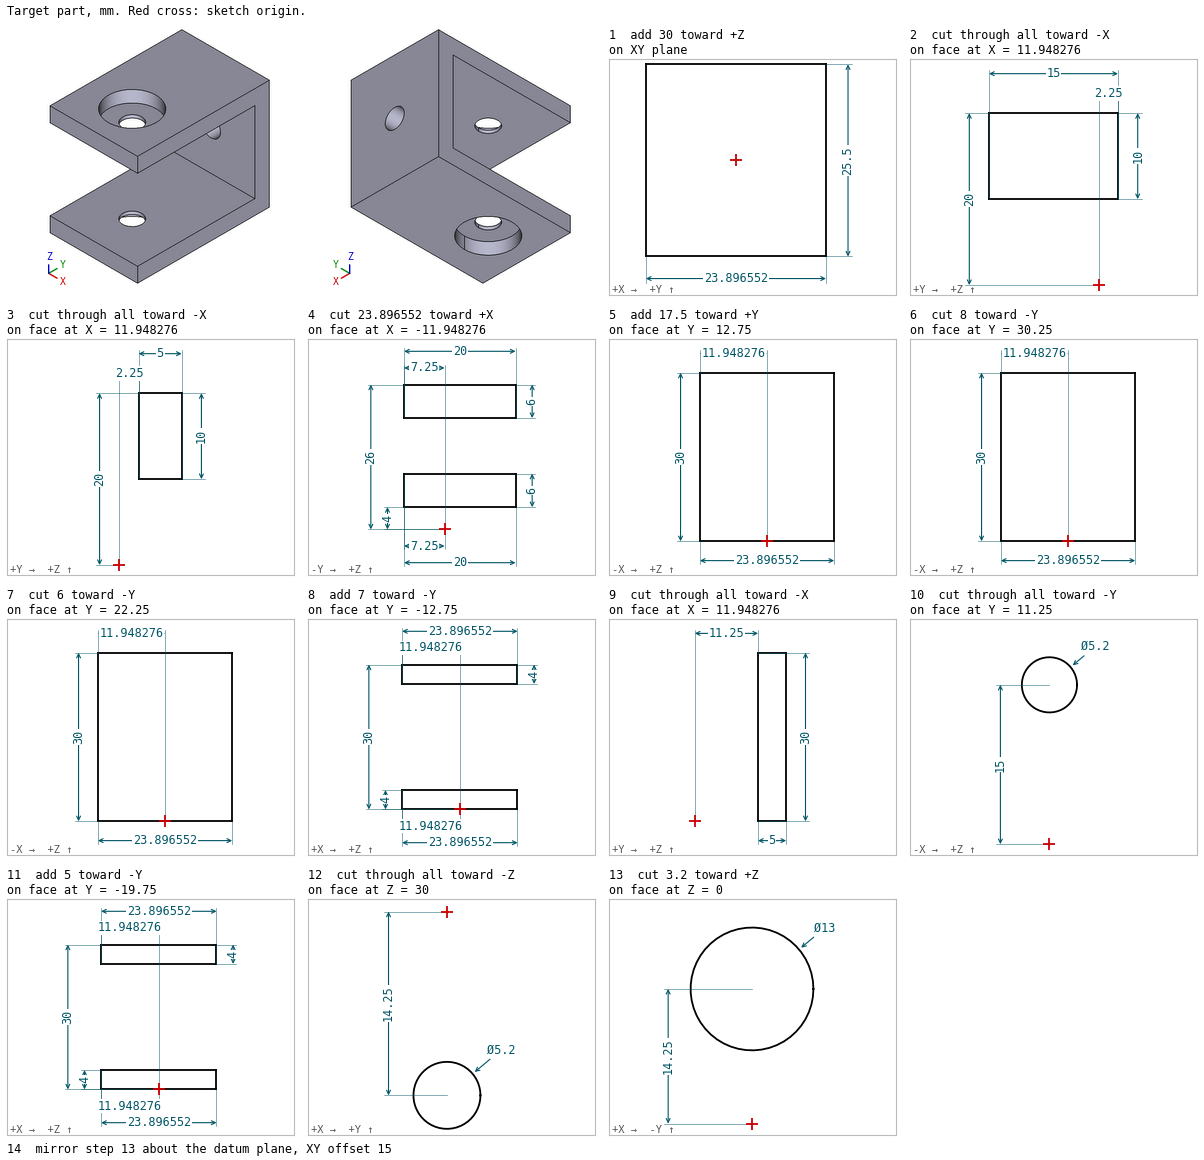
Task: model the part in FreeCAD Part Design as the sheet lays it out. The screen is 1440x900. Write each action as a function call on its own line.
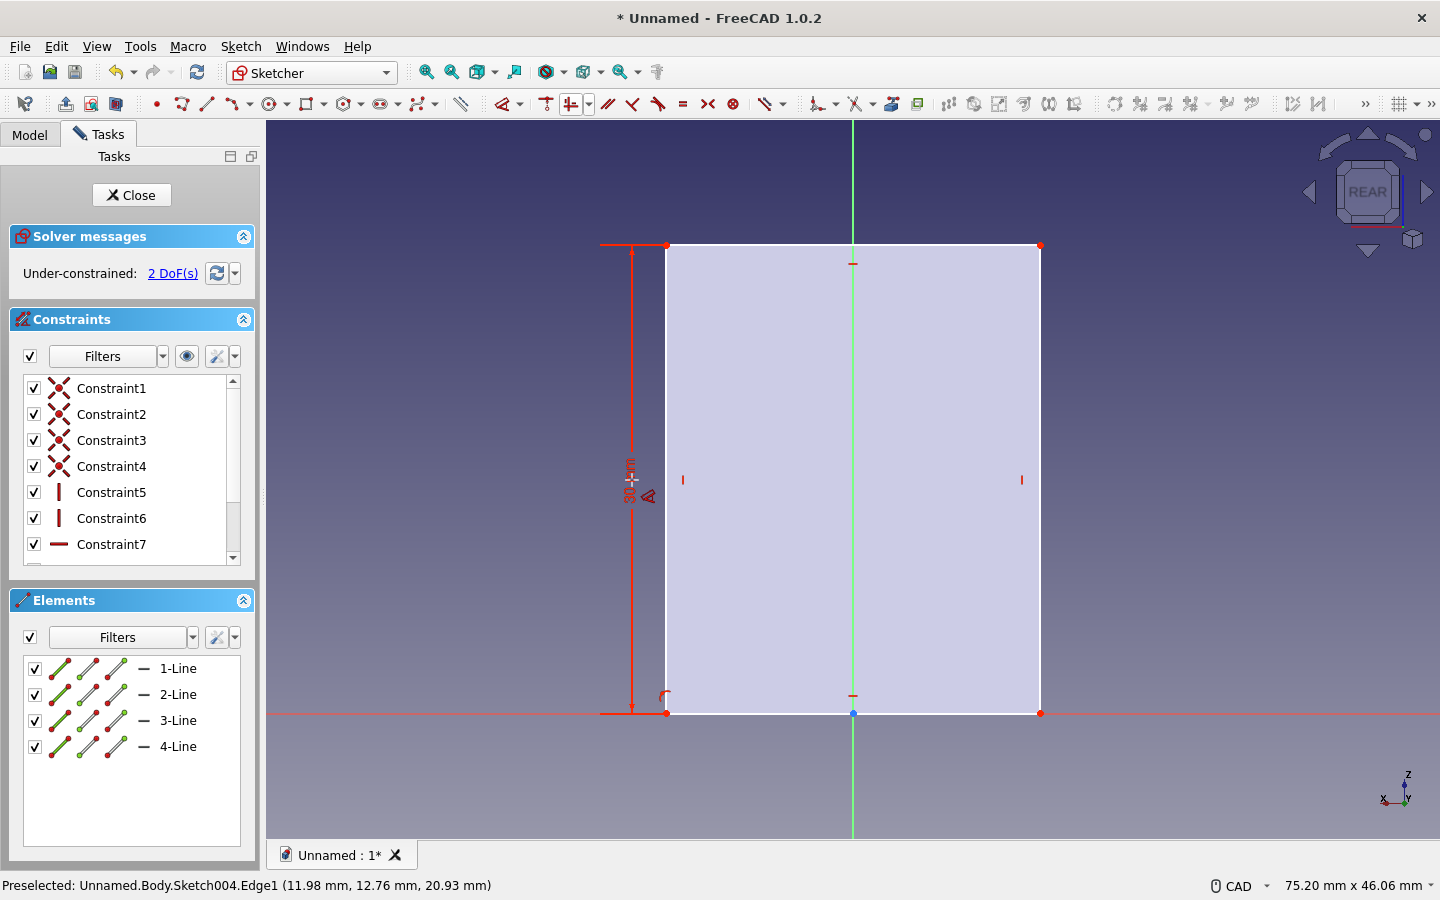
click(778, 714)
click(767, 748)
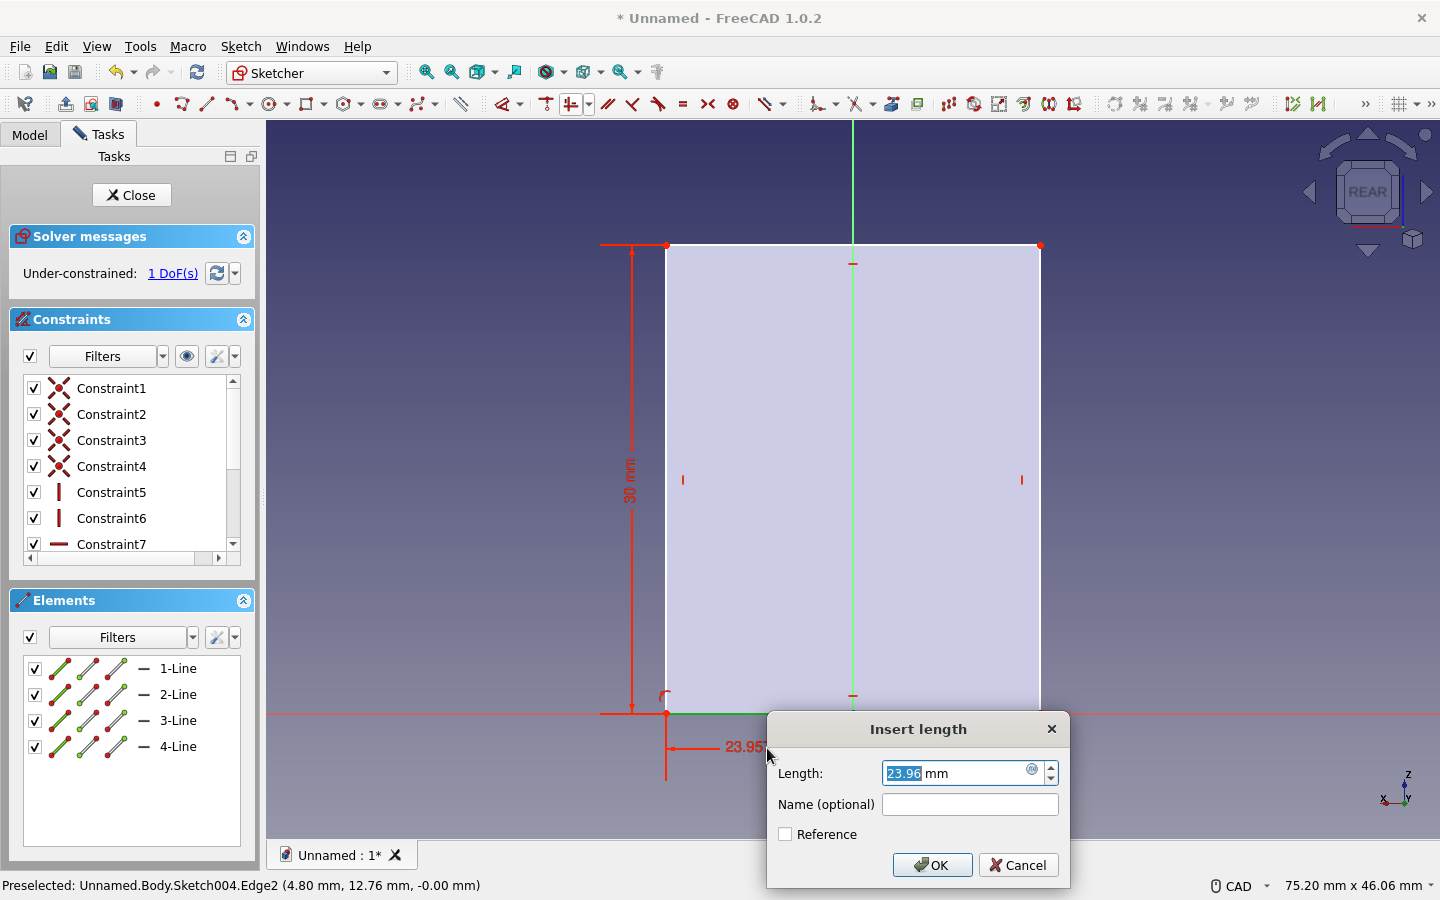
text(23.896552)
key(Return)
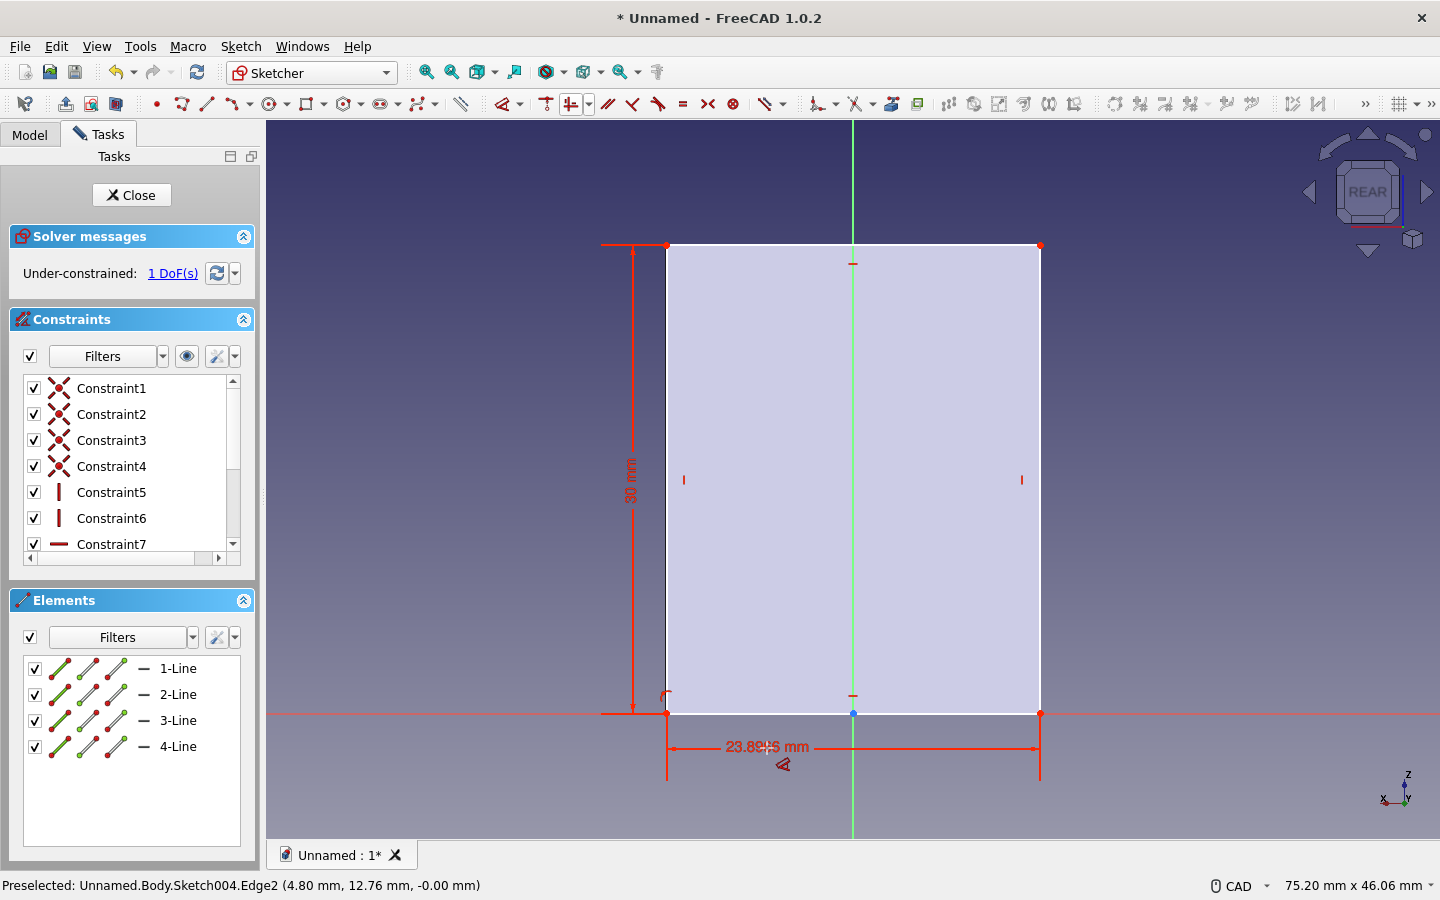
click(667, 245)
click(695, 748)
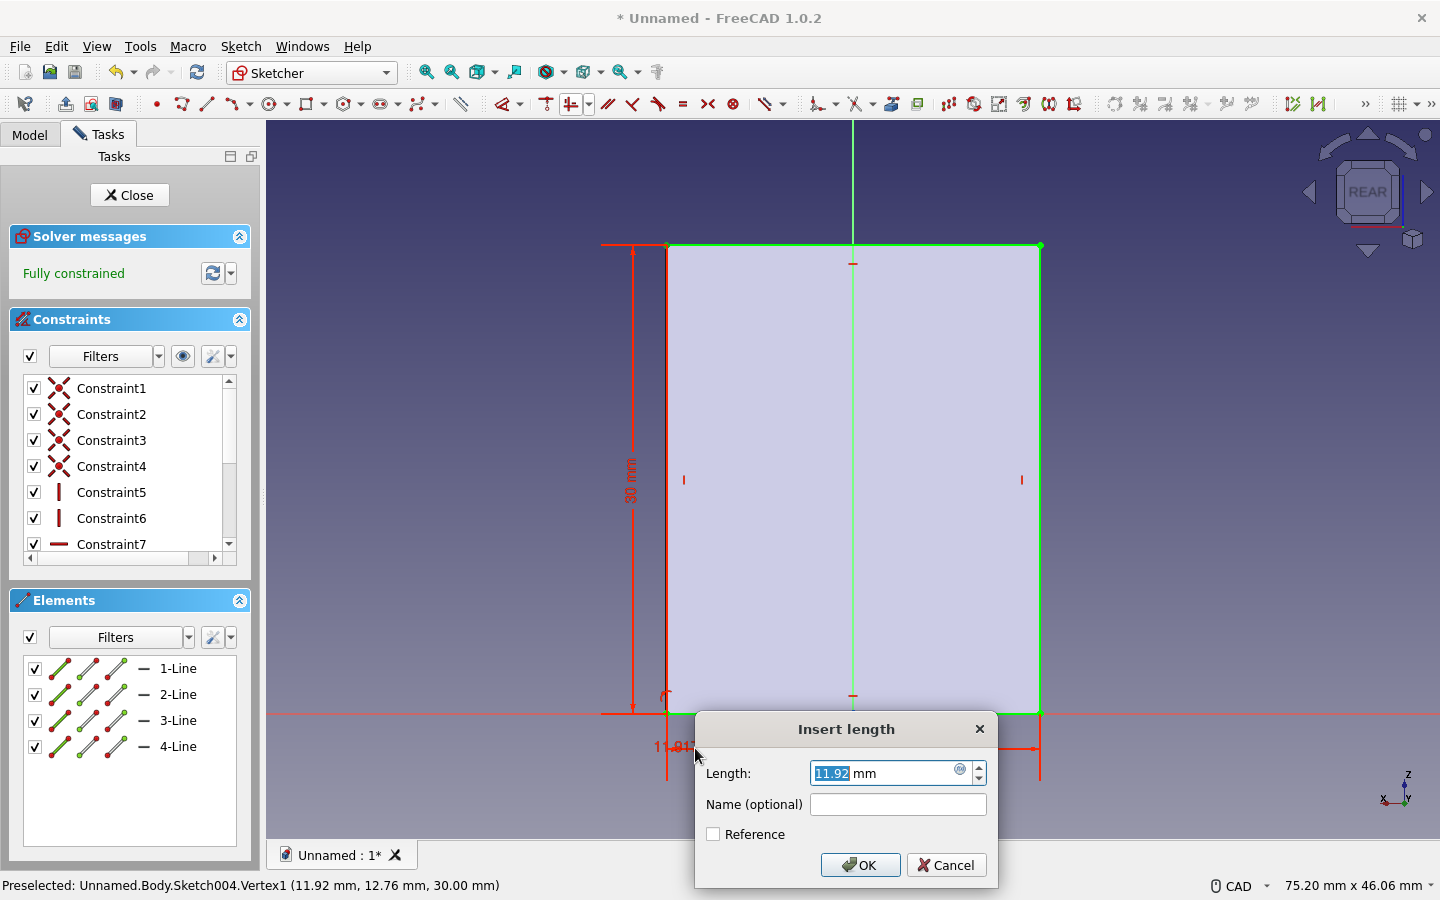
text(11.948276)
key(Return)
key(Escape)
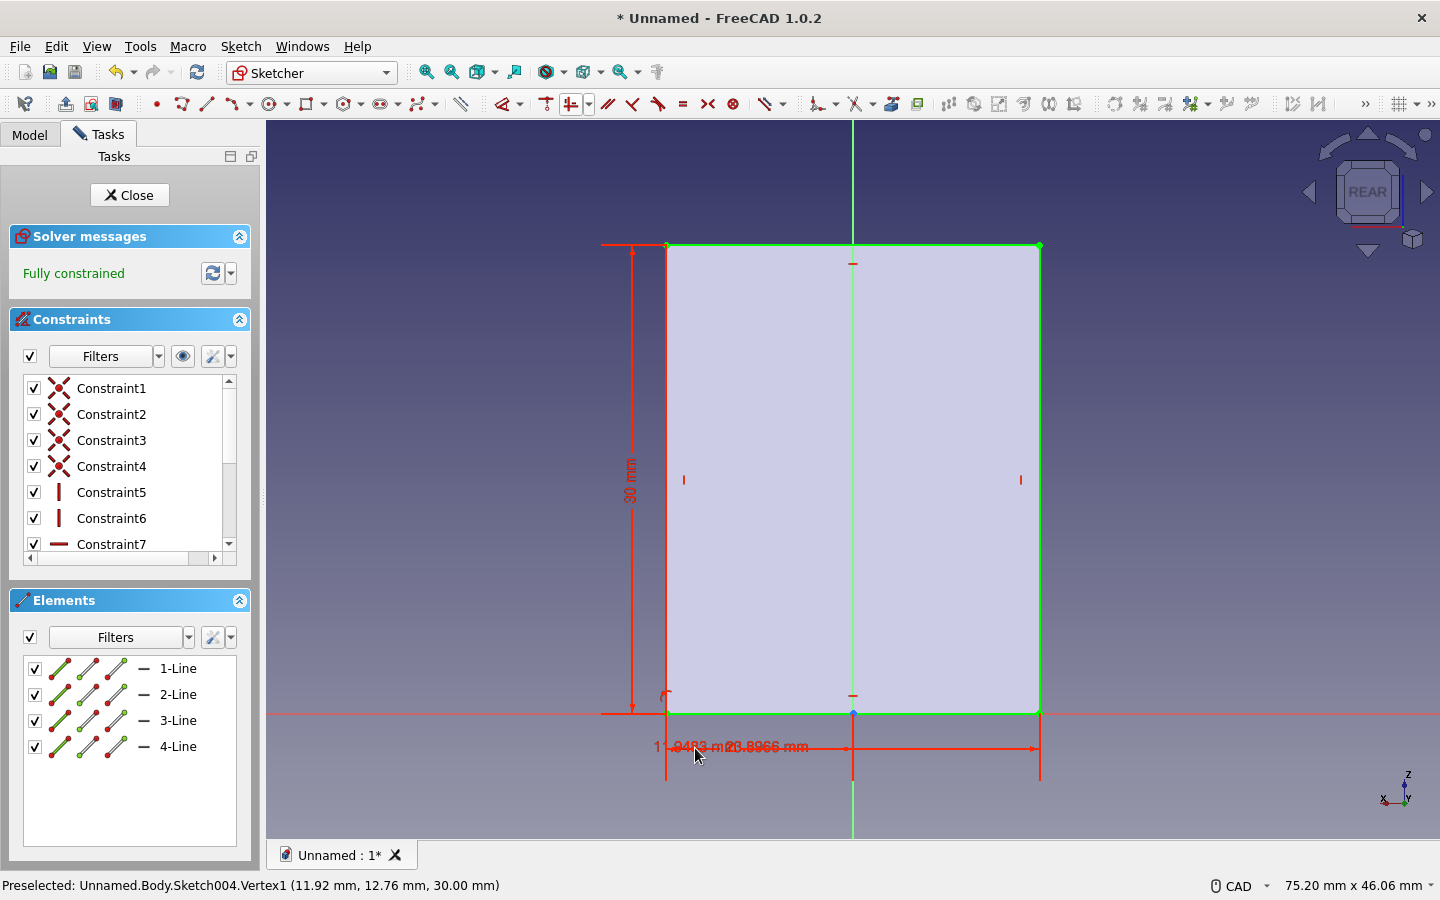
click(130, 195)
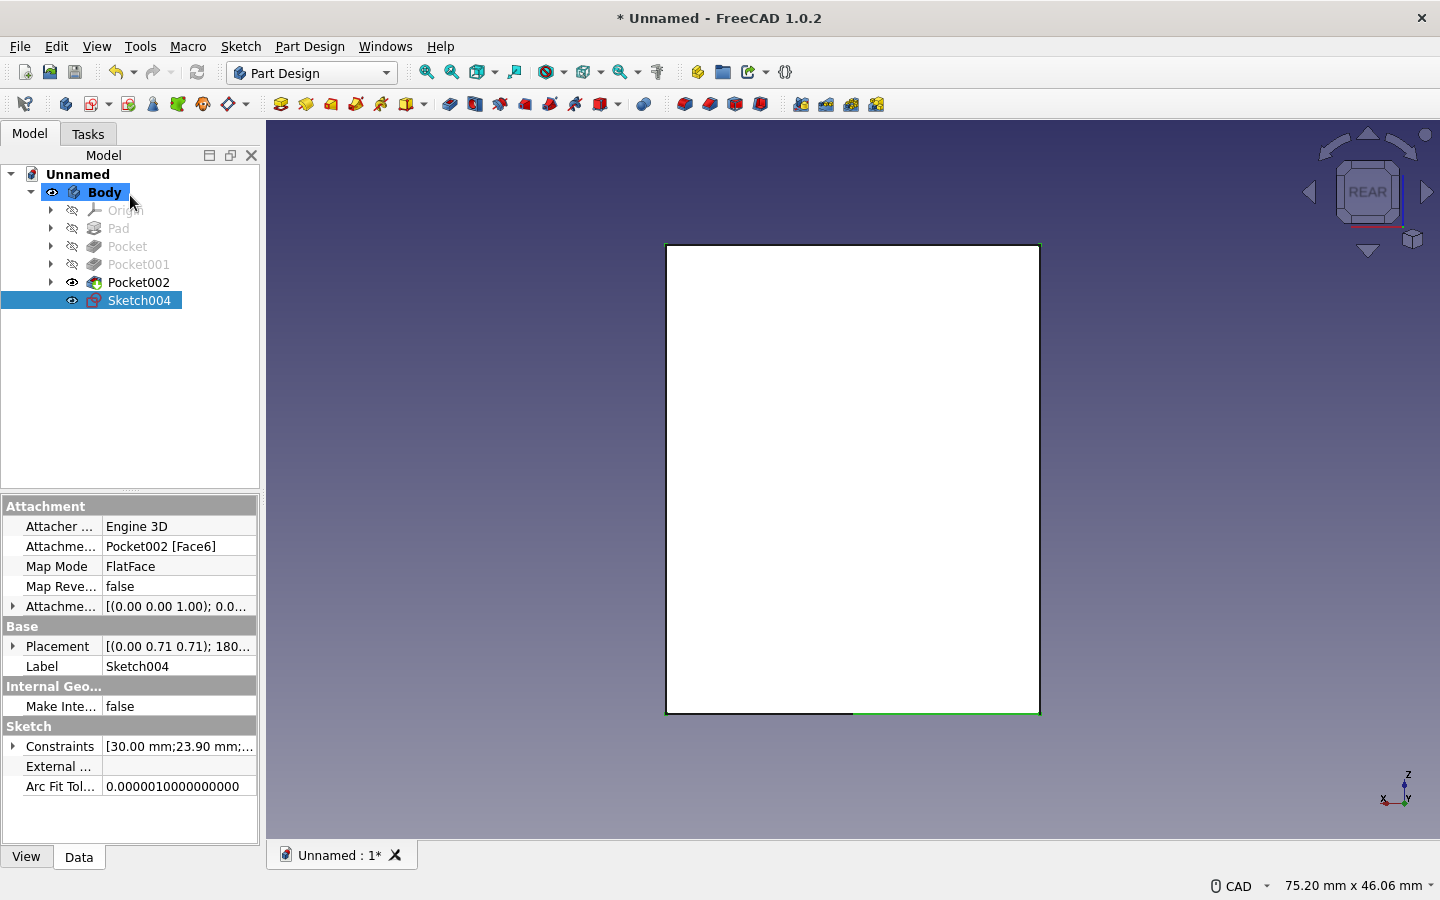
click(281, 104)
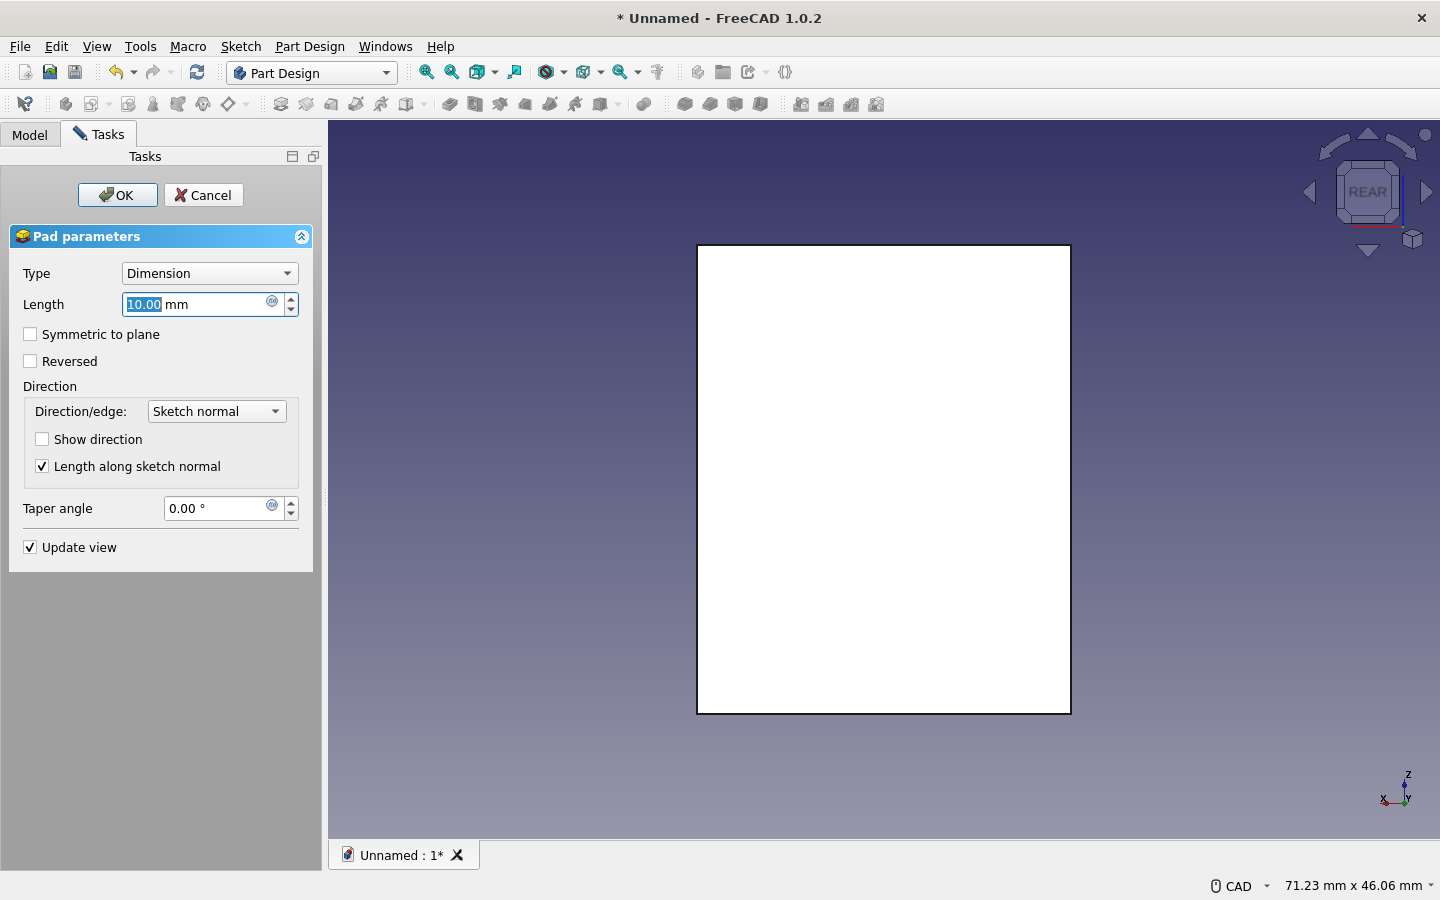
text(17.5)
key(Tab)